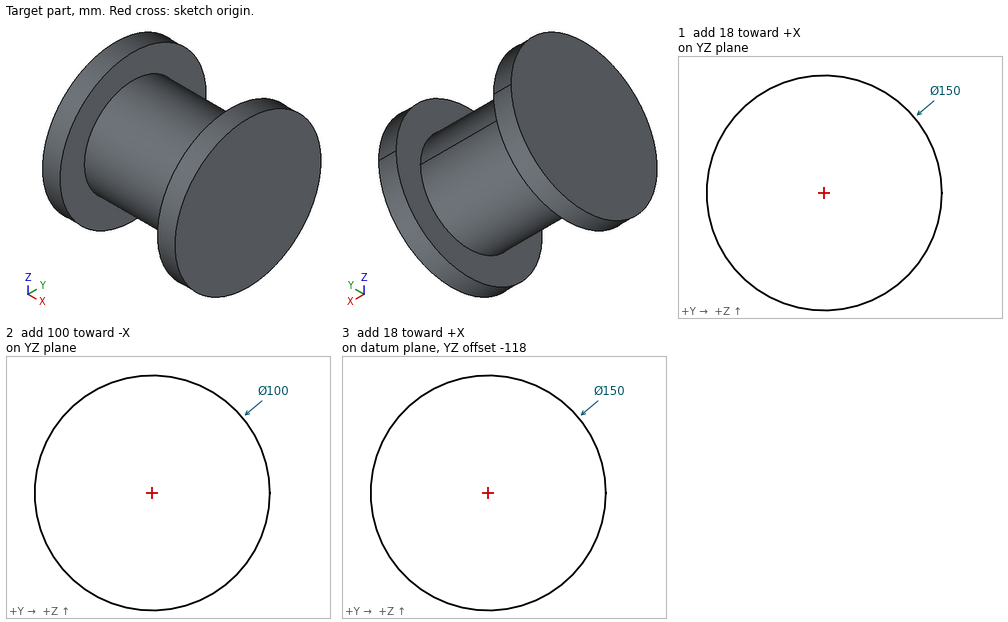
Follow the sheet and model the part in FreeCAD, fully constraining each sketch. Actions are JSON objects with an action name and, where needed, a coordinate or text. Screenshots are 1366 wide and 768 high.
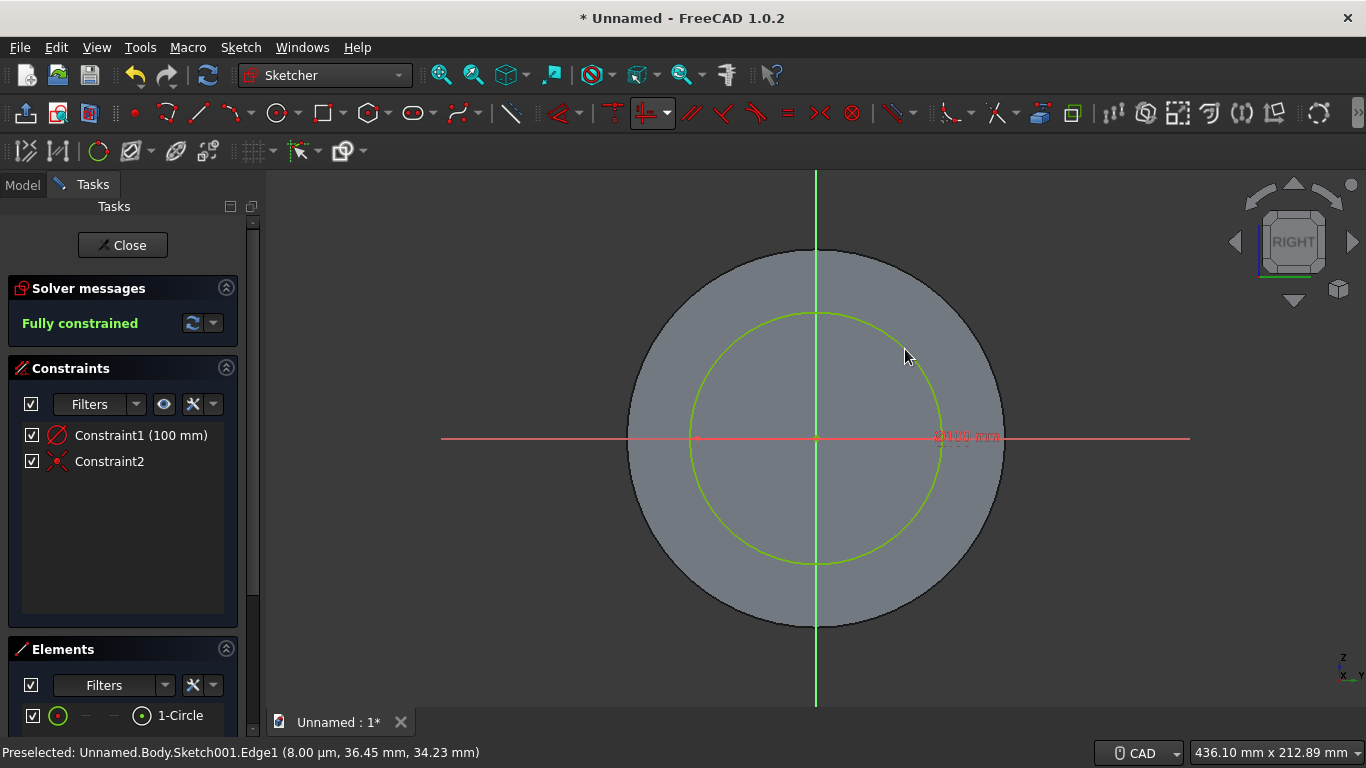
{"action": "left_click", "coordinate": [123, 245]}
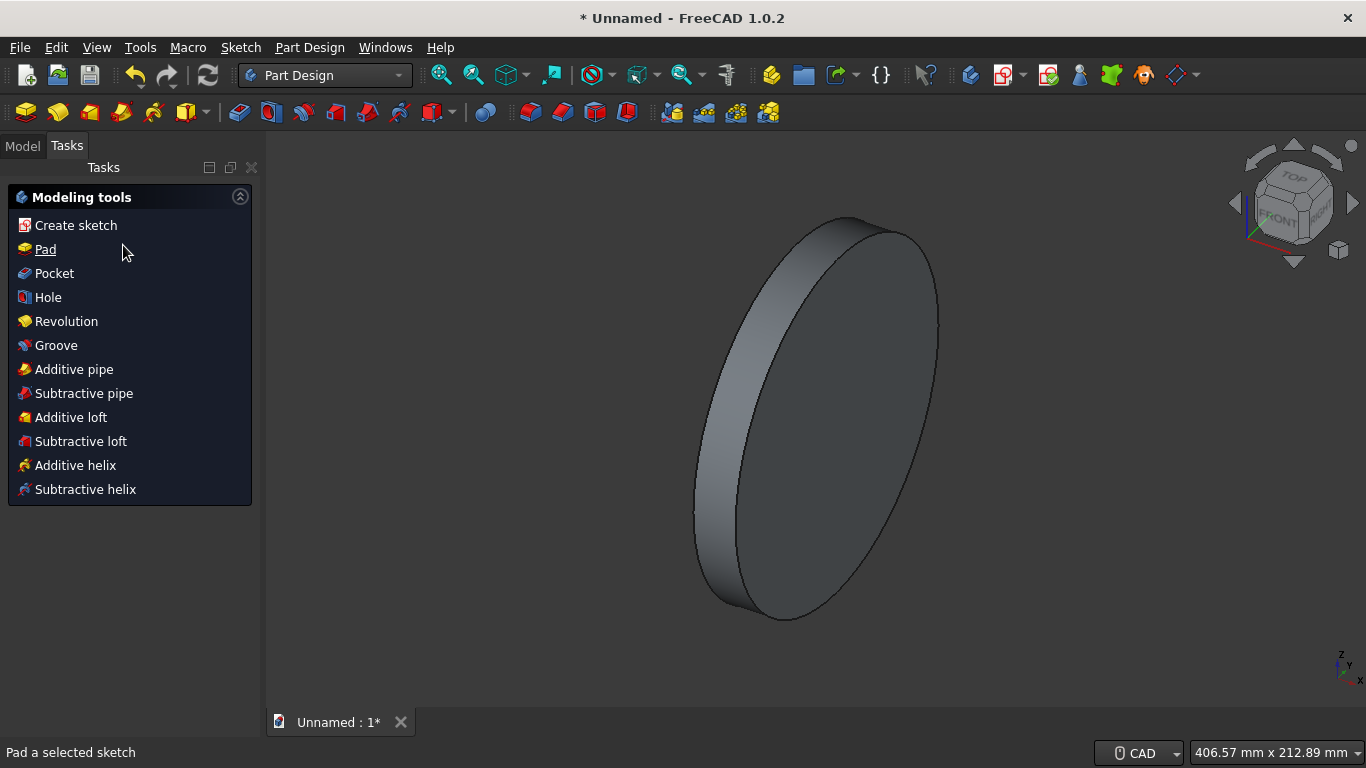
{"action": "left_click", "coordinate": [26, 112]}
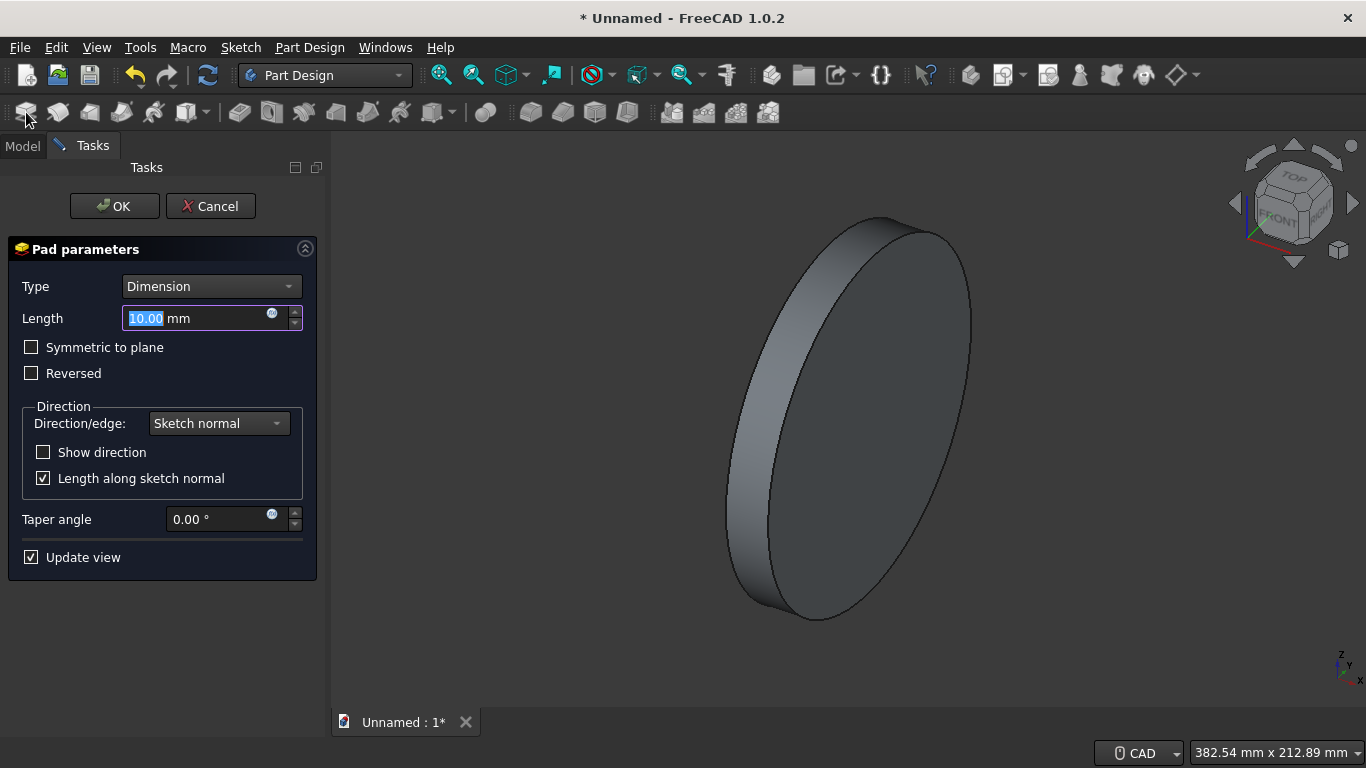
{"action": "type", "text": "100"}
{"action": "key", "text": "Tab"}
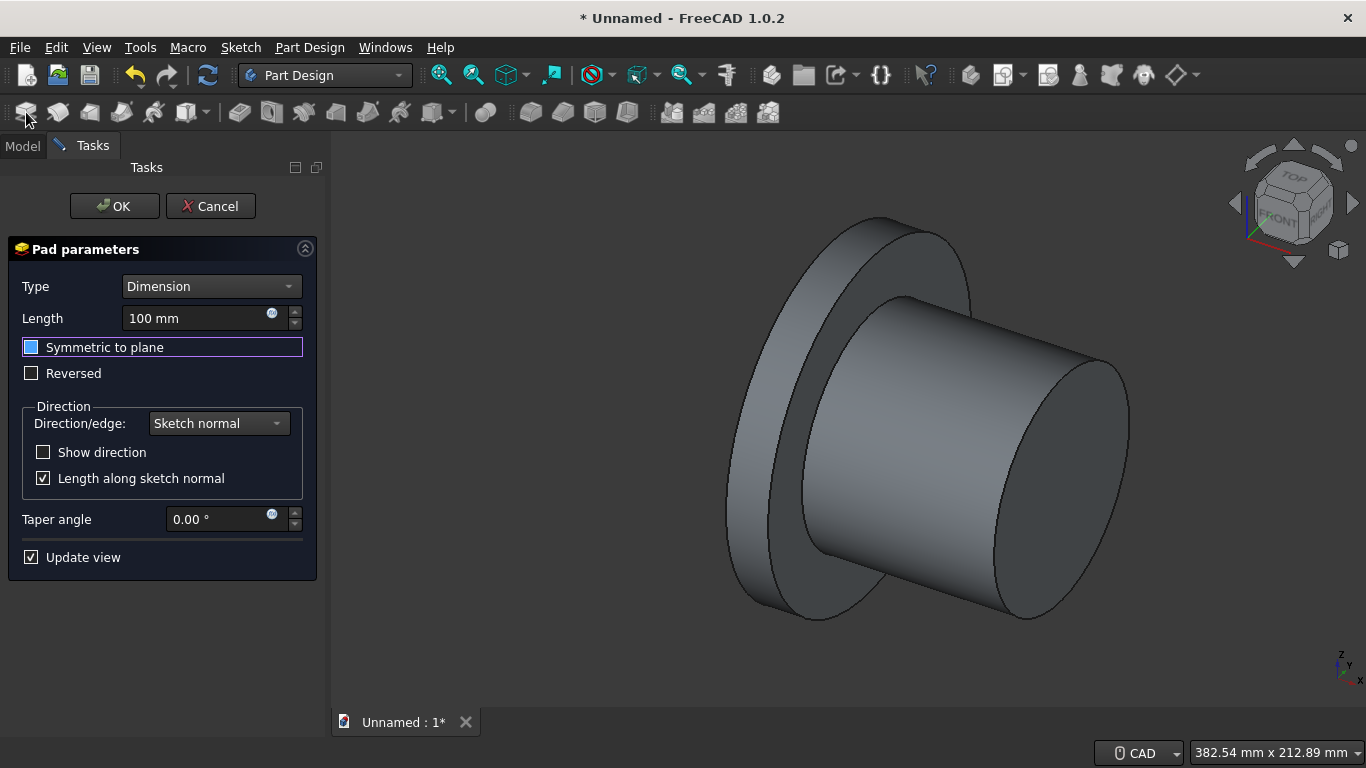
{"action": "left_click", "coordinate": [30, 373]}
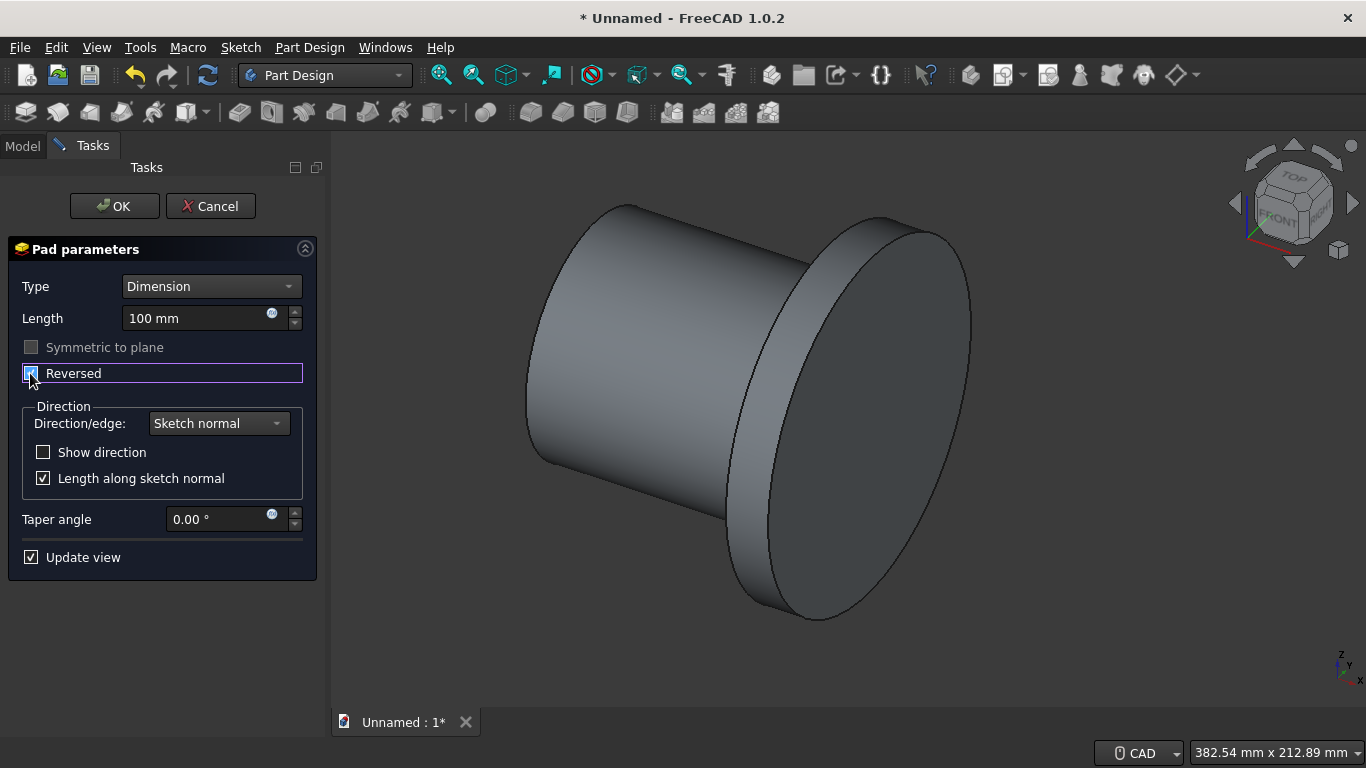
{"action": "left_click", "coordinate": [115, 206]}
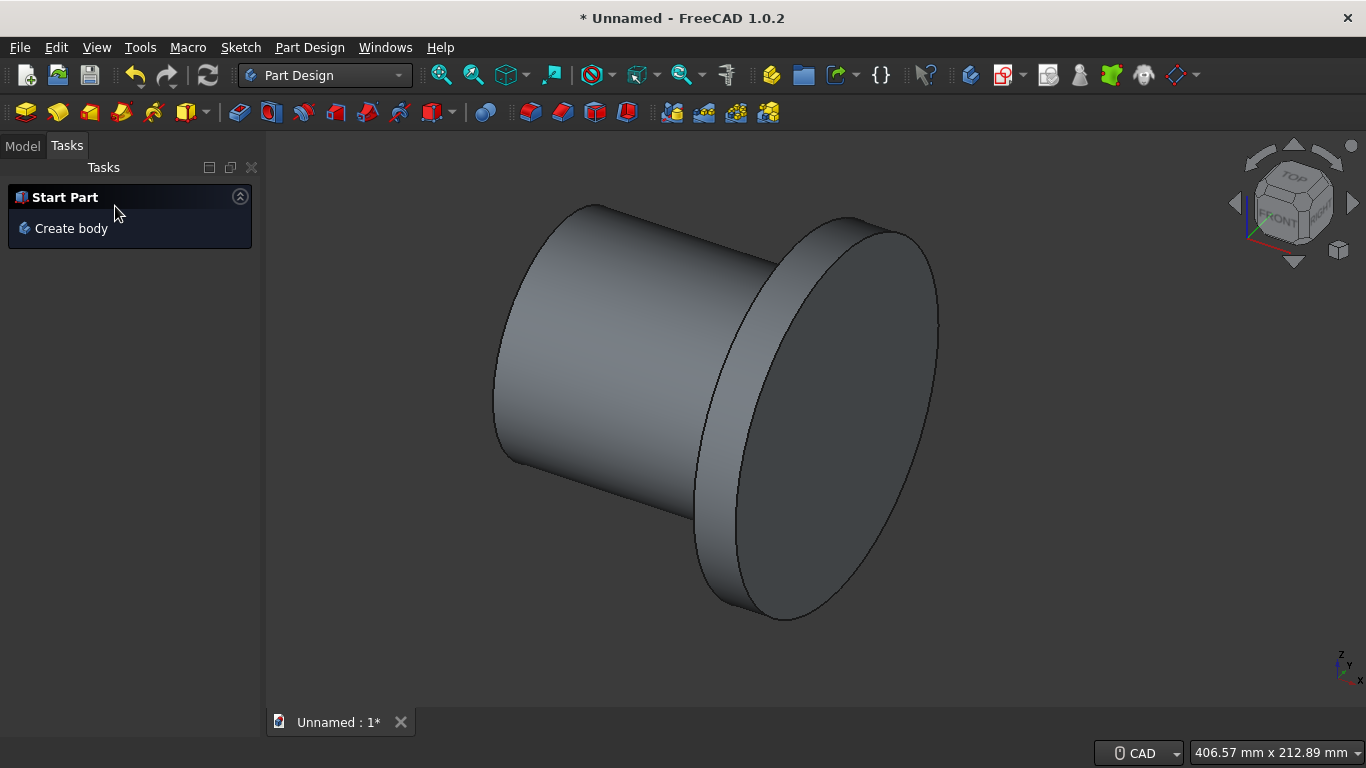
{"action": "left_click", "coordinate": [442, 76]}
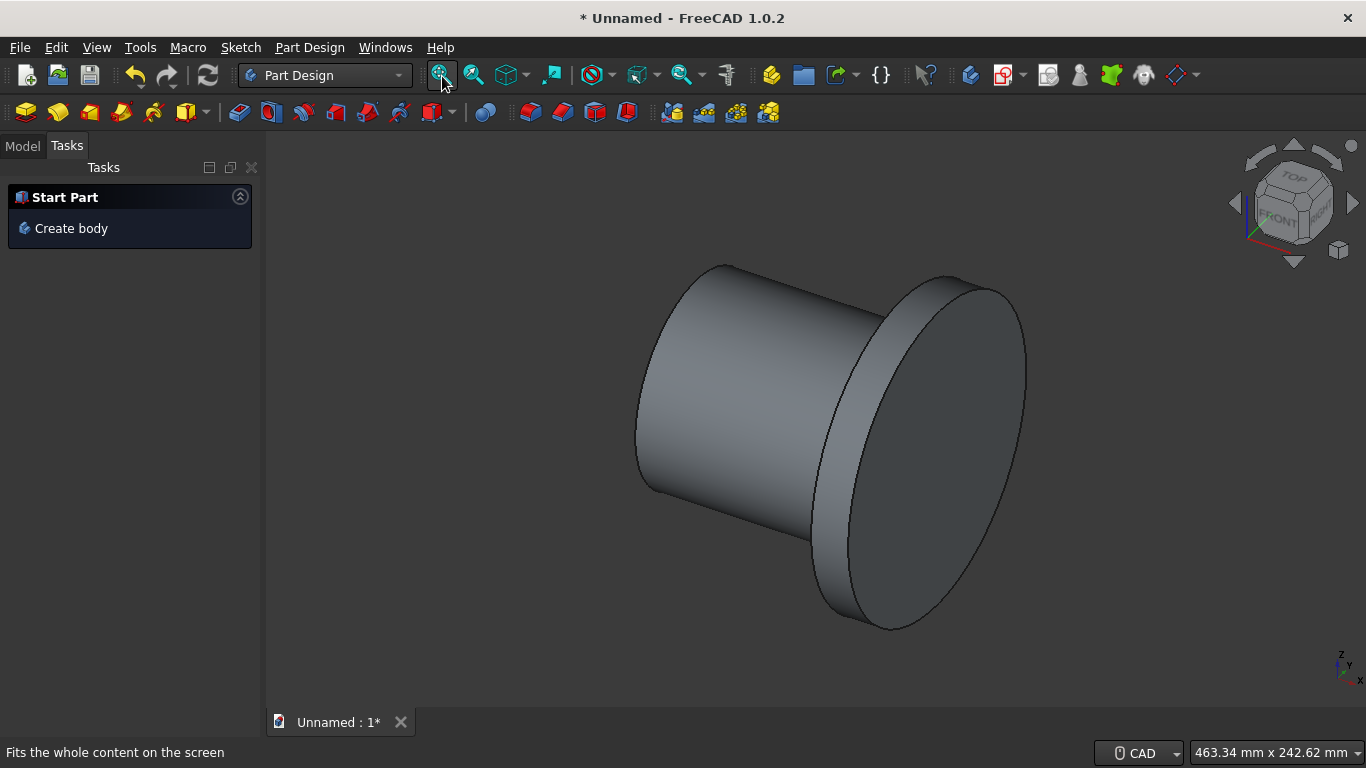
{"action": "left_click", "coordinate": [23, 145]}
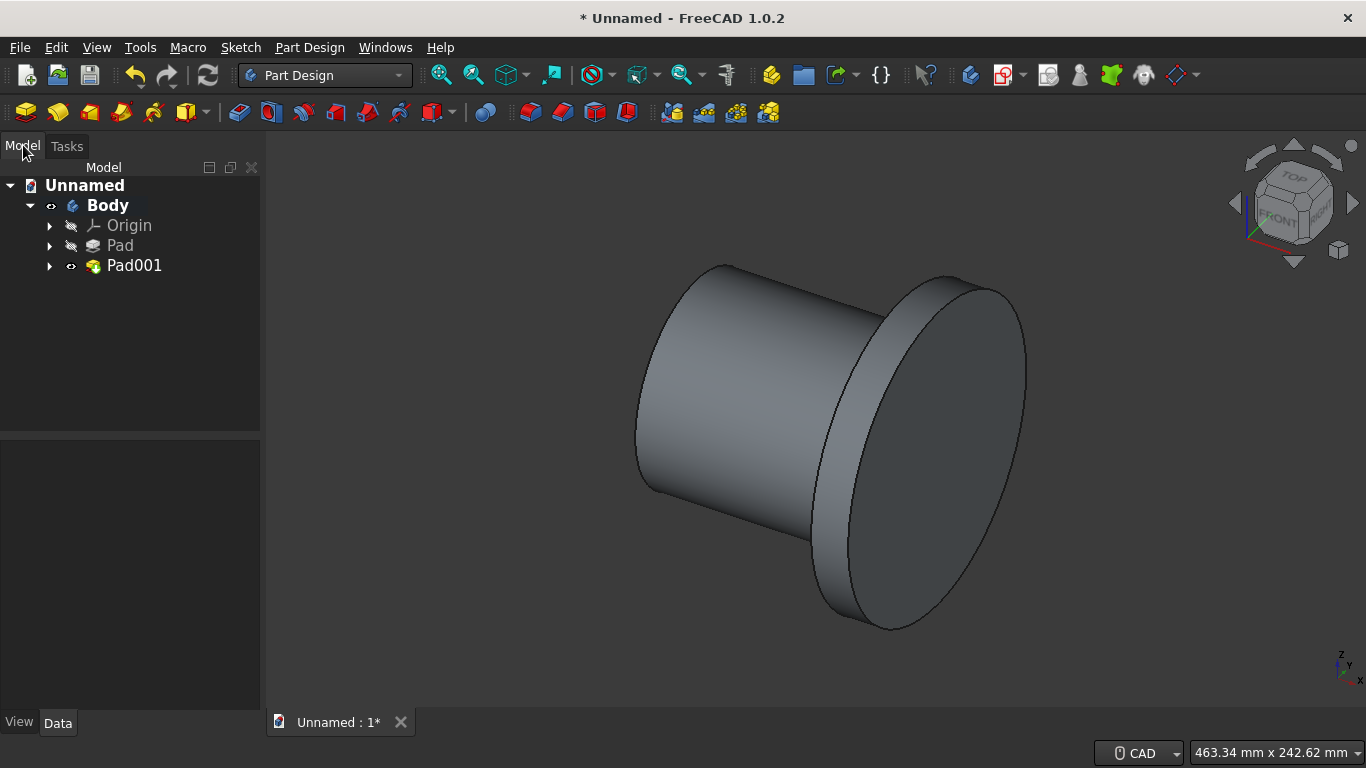
{"action": "left_click", "coordinate": [50, 226]}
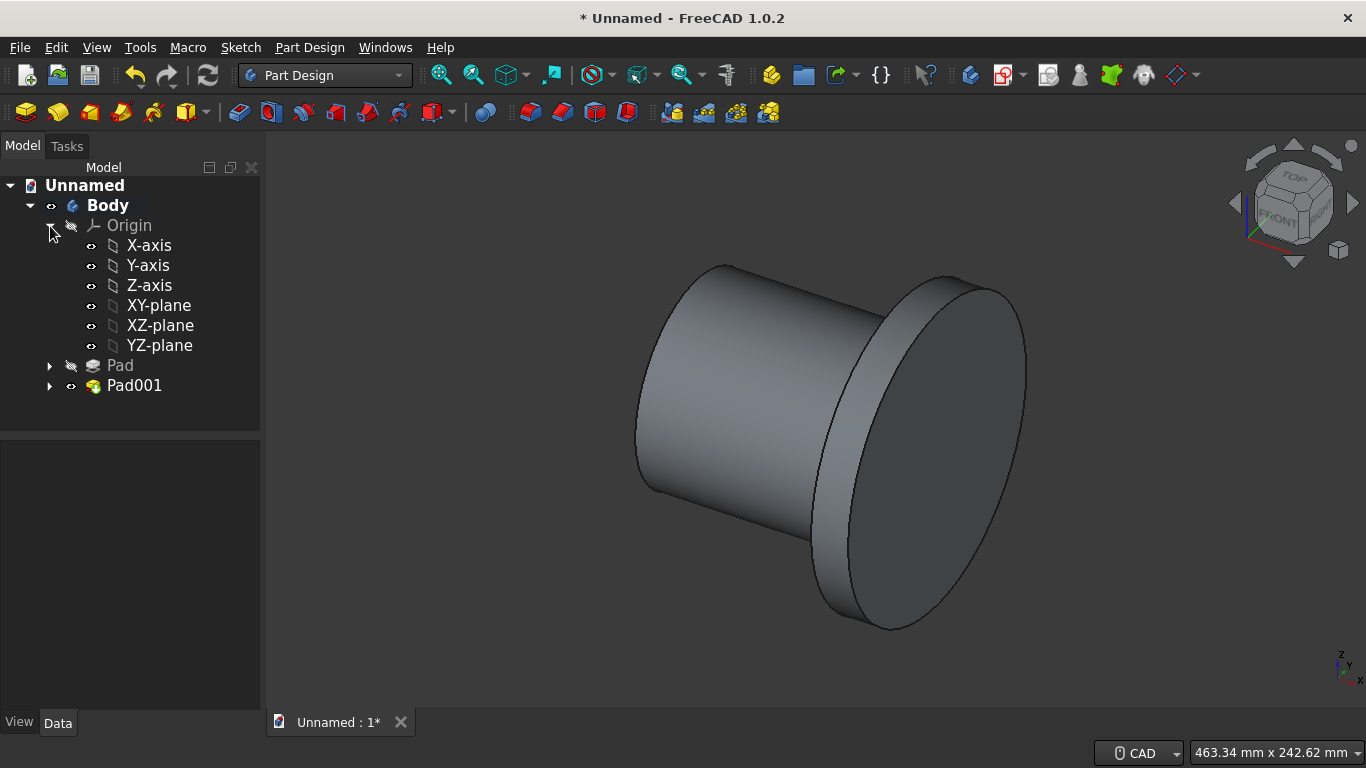
{"action": "left_click", "coordinate": [136, 346]}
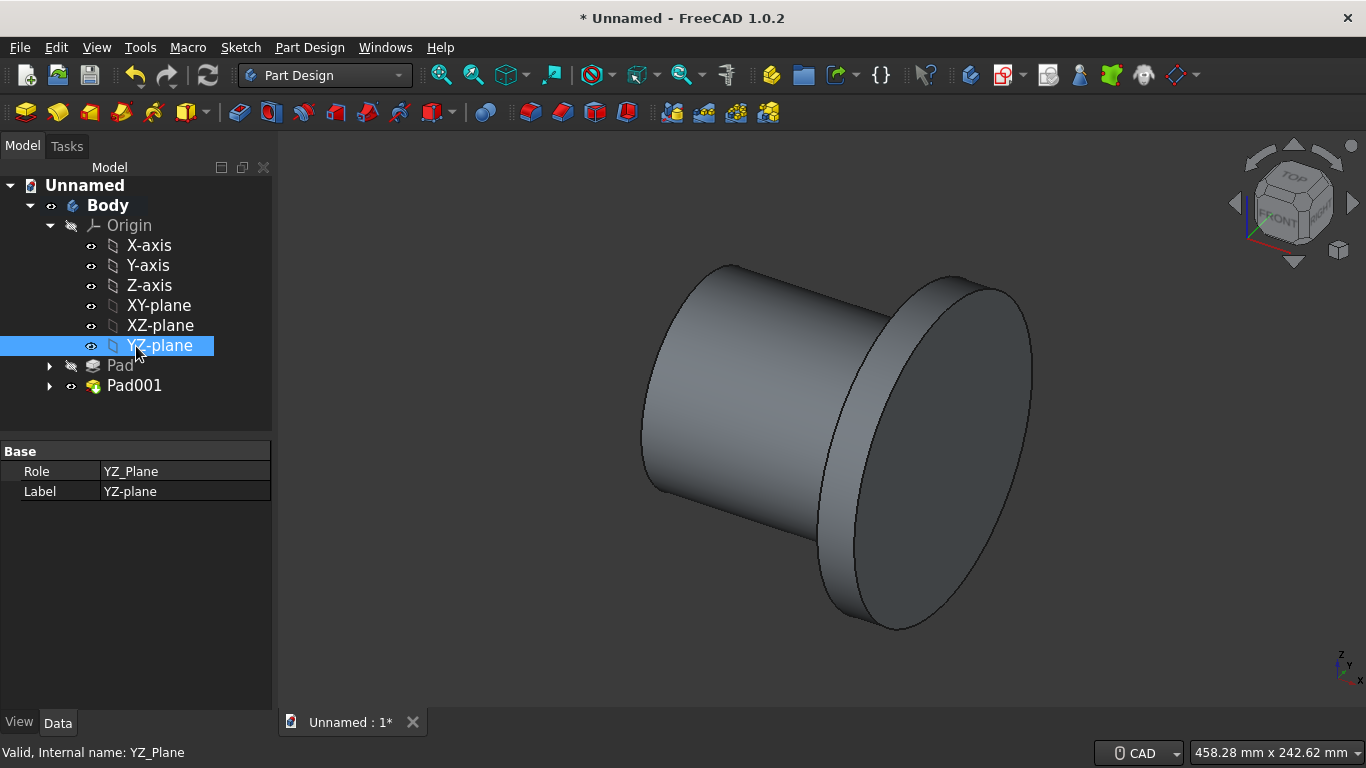
{"action": "left_click", "coordinate": [1176, 76]}